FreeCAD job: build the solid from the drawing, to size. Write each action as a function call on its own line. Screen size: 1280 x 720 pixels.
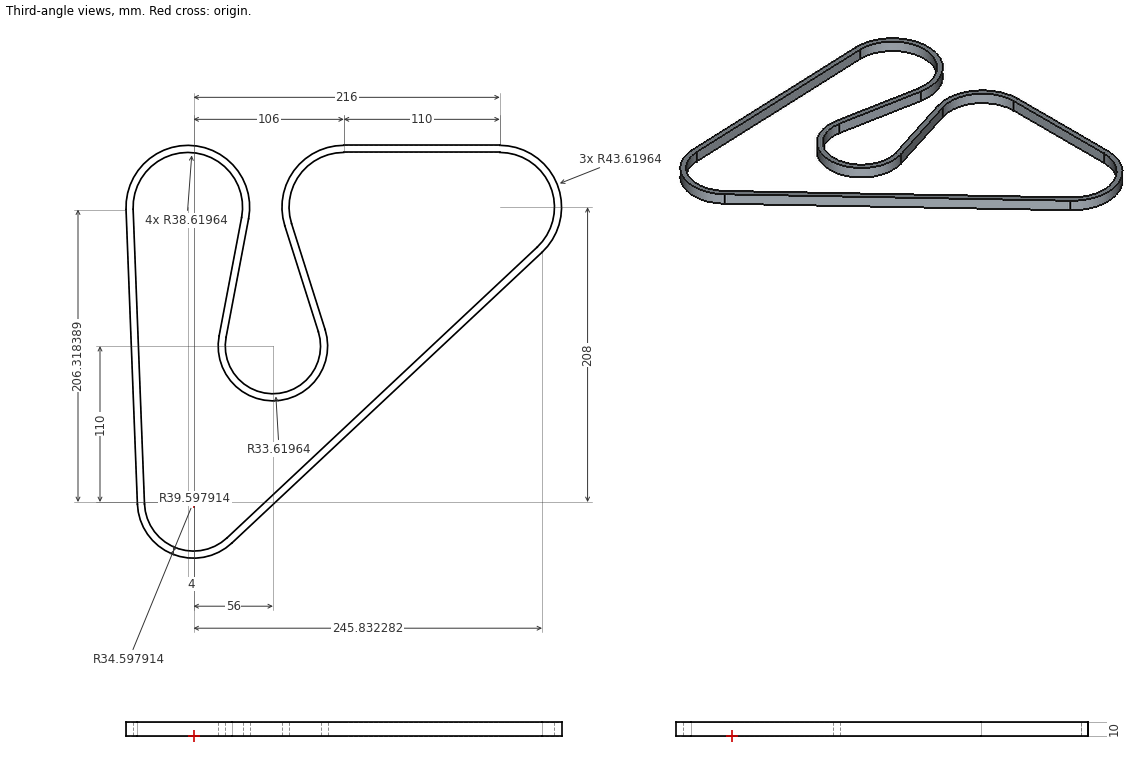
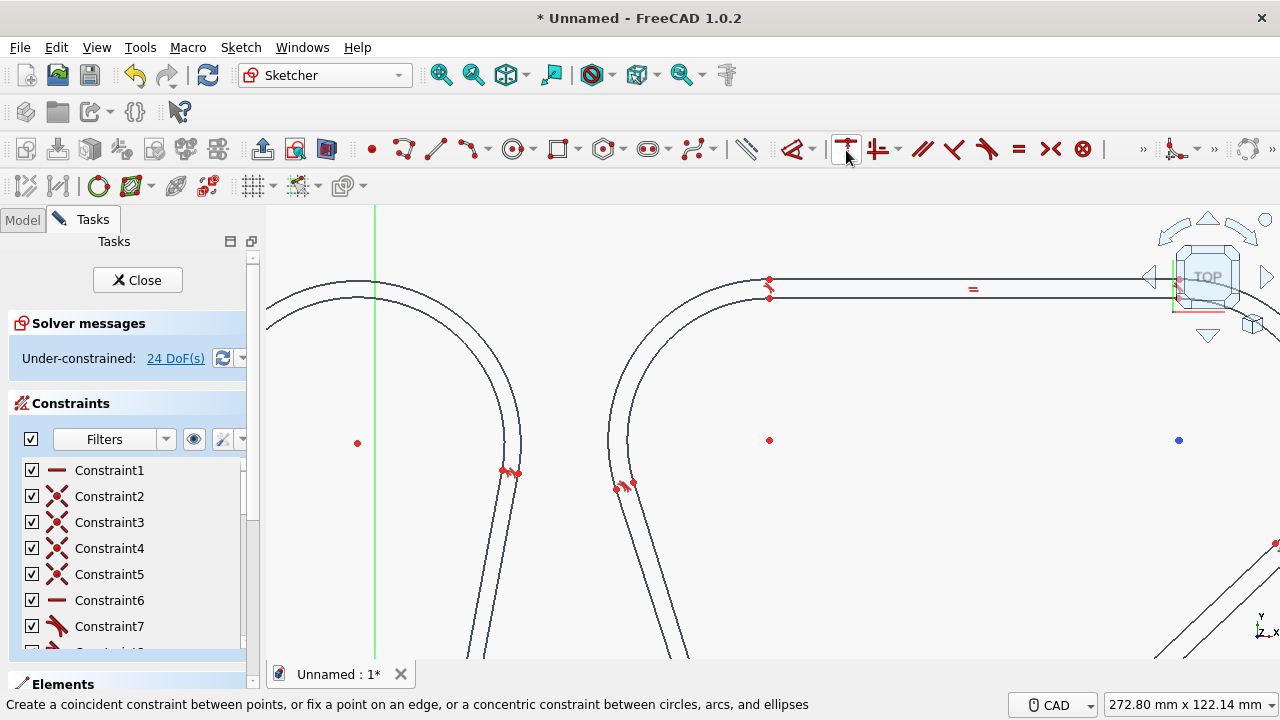
scroll(685, 308, down, 7)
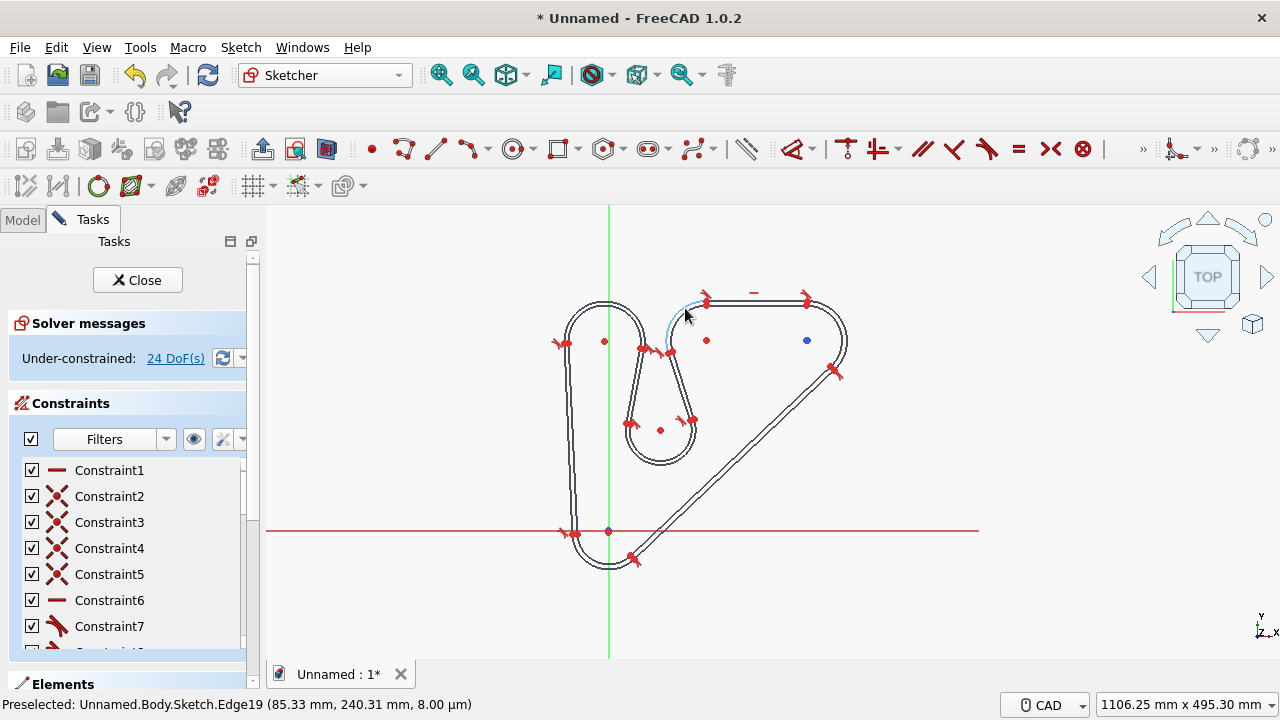
scroll(847, 345, up, 6)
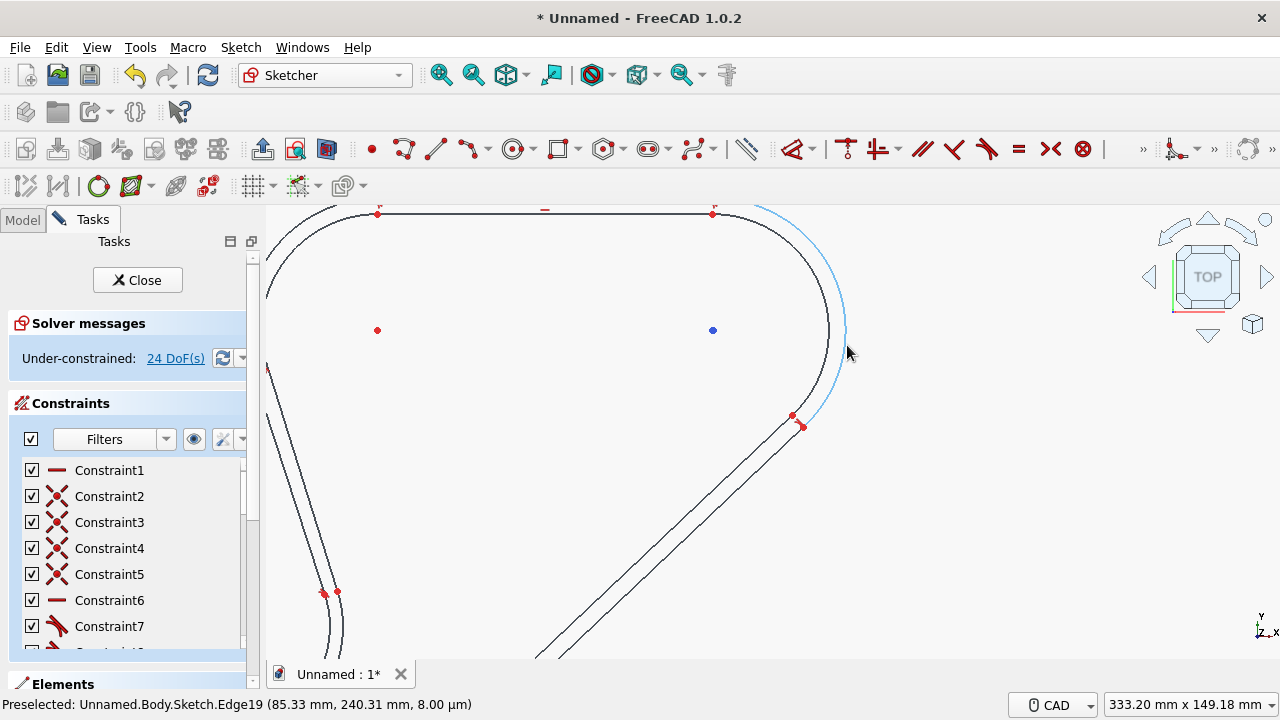
click(845, 344)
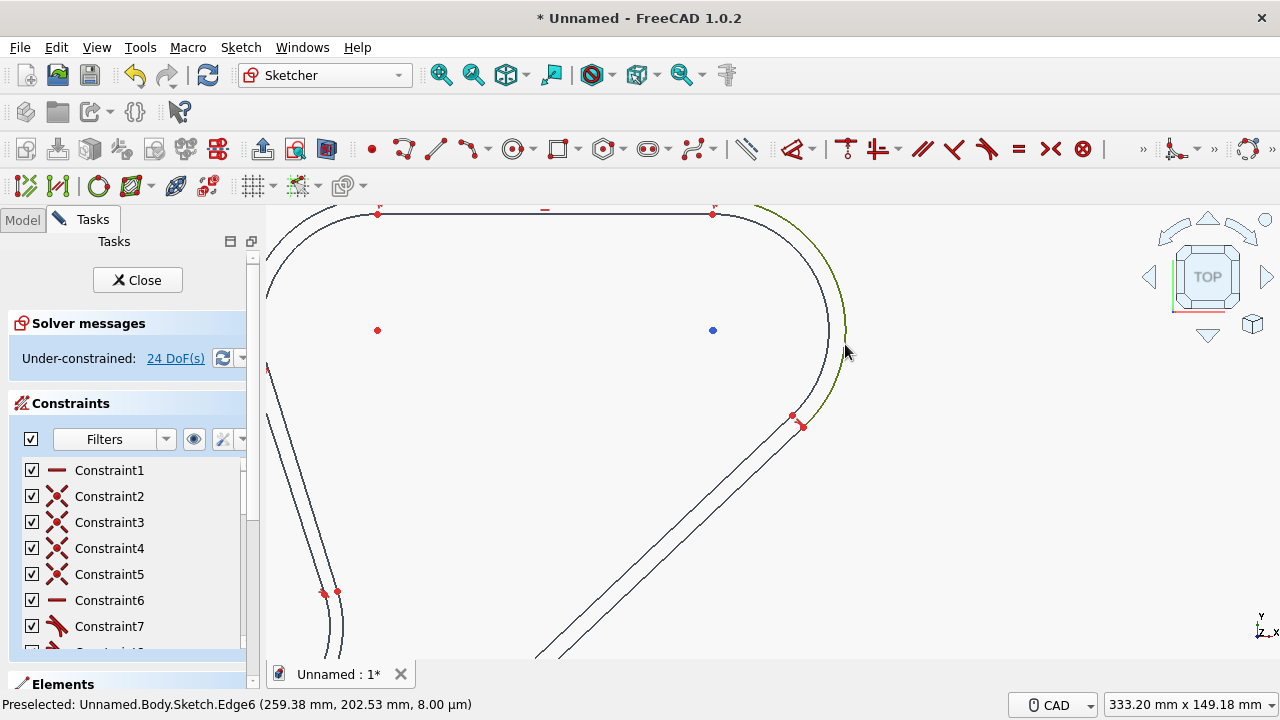
click(828, 342)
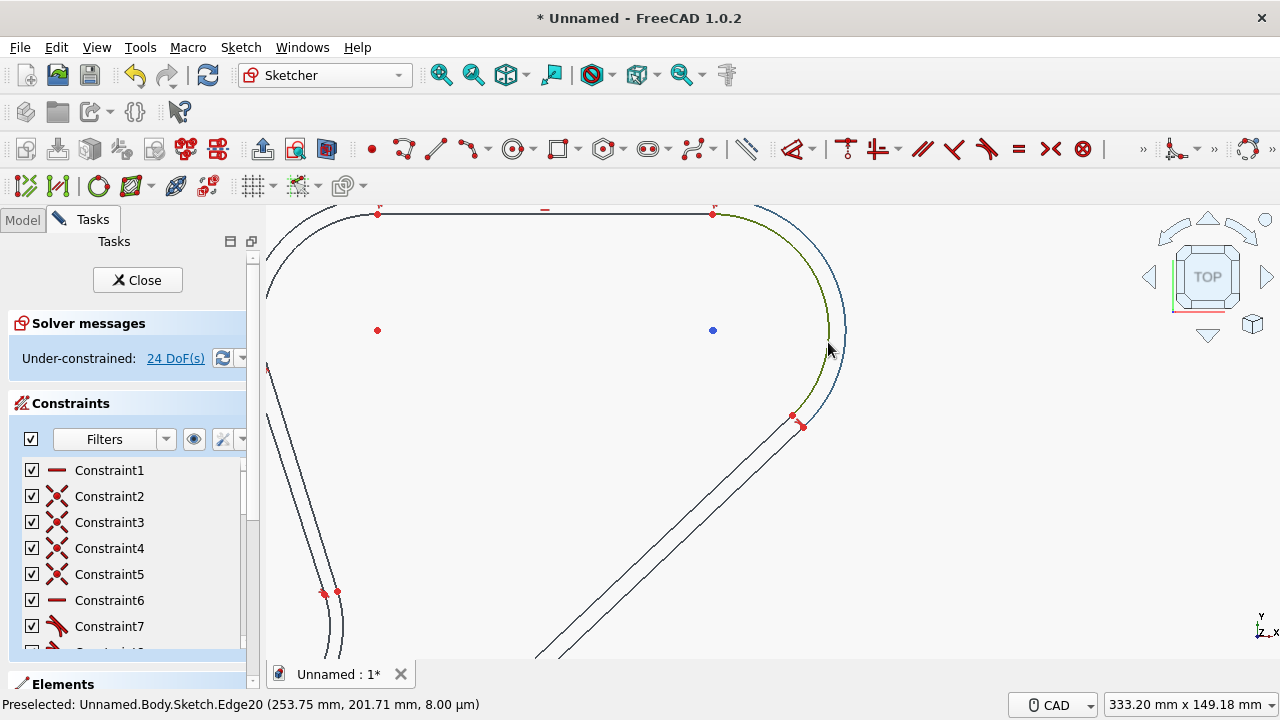
click(846, 150)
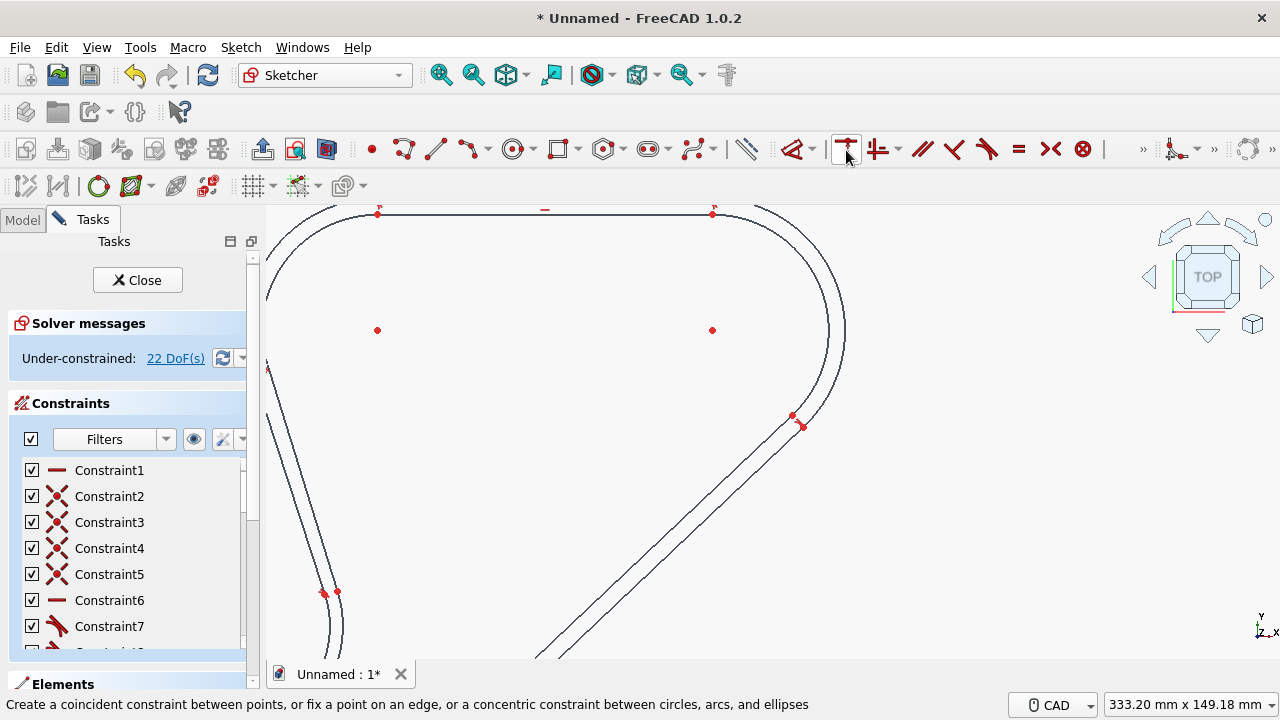
scroll(847, 345, down, 6)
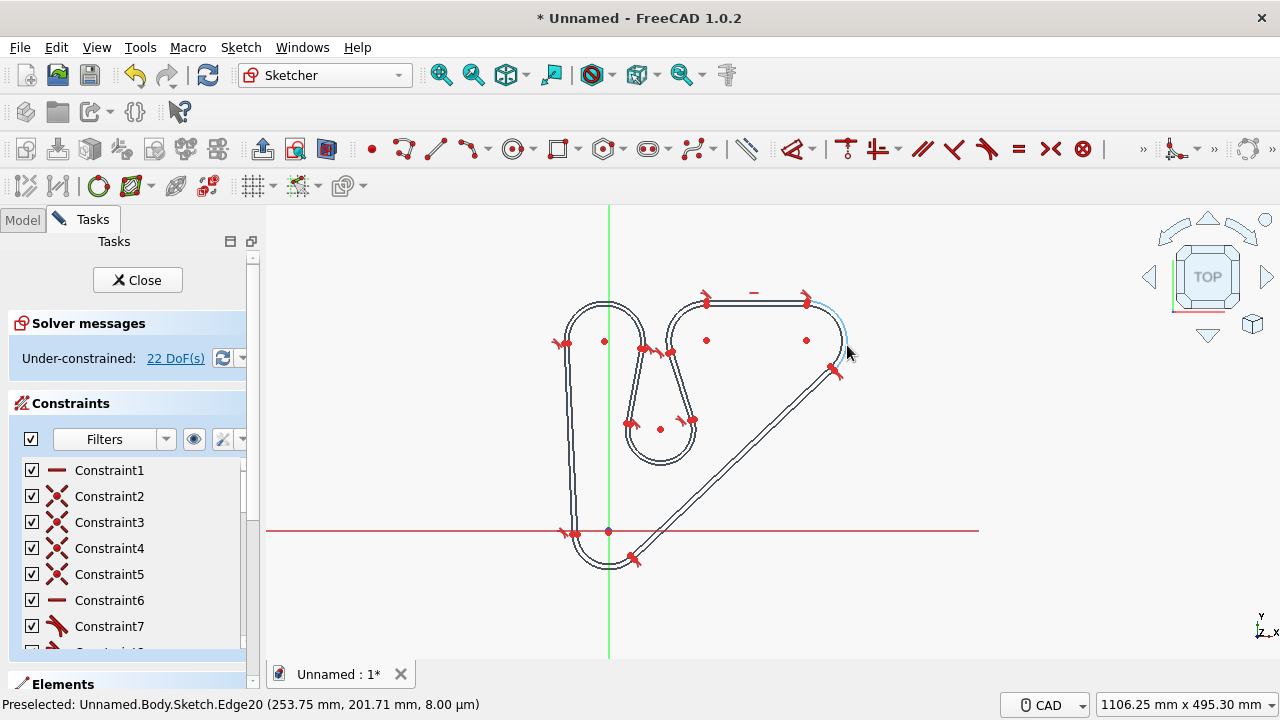
scroll(609, 532, up, 2)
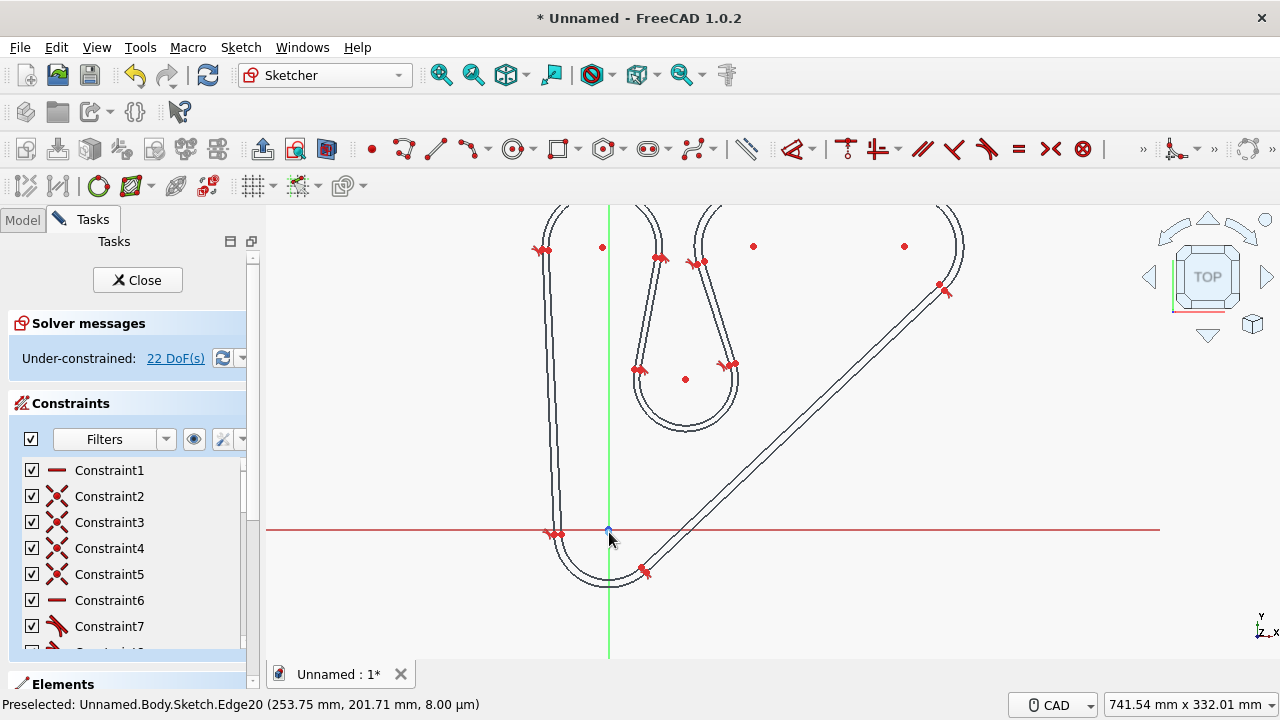
drag(599, 520, 619, 543)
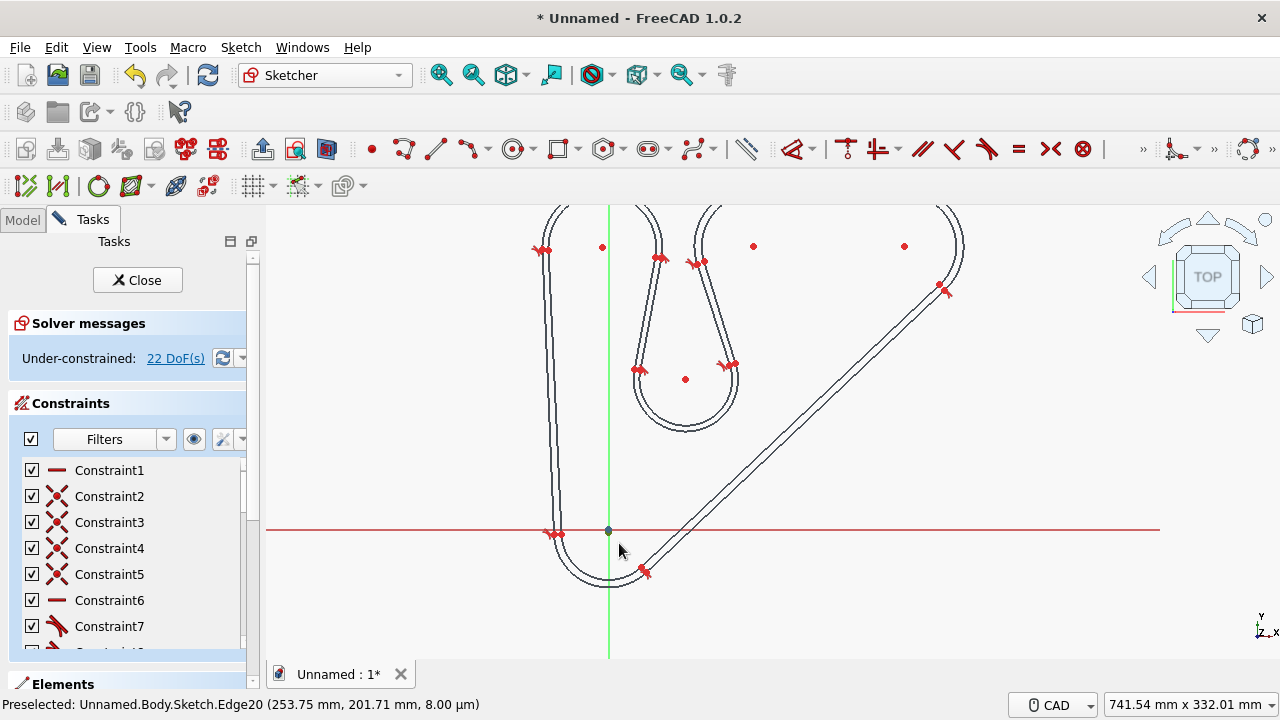
click(846, 150)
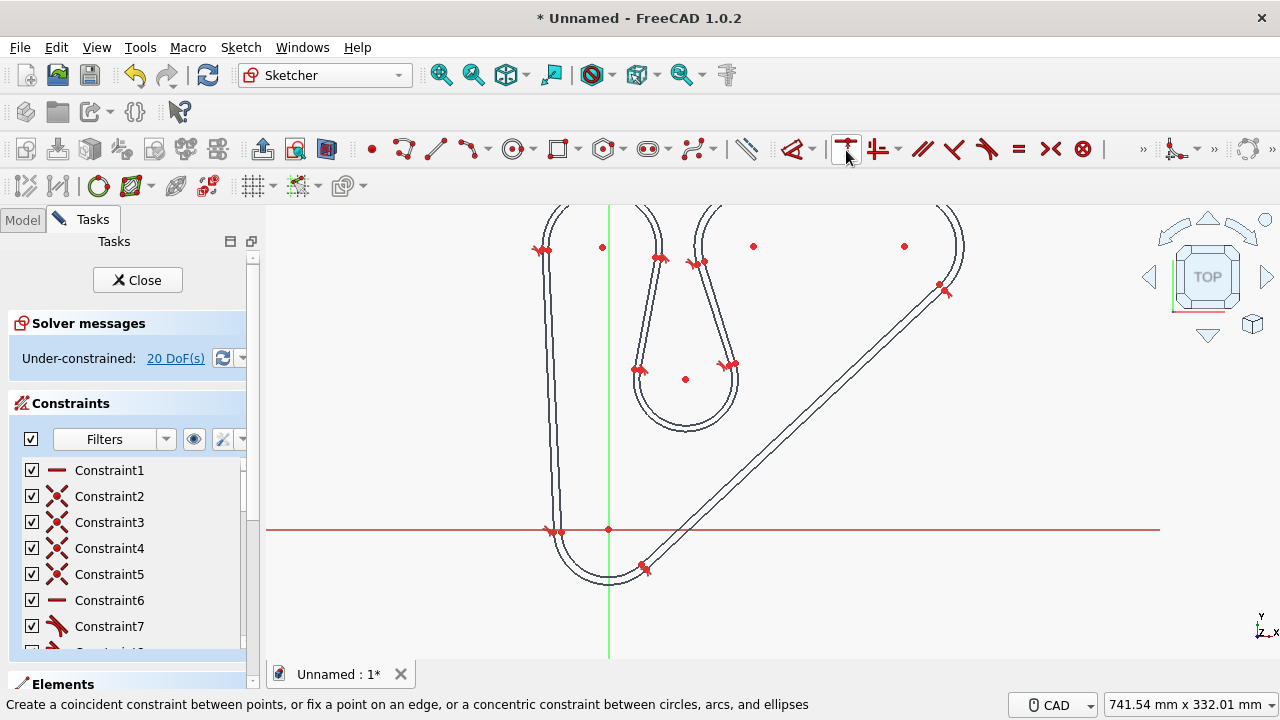
scroll(609, 532, down, 2)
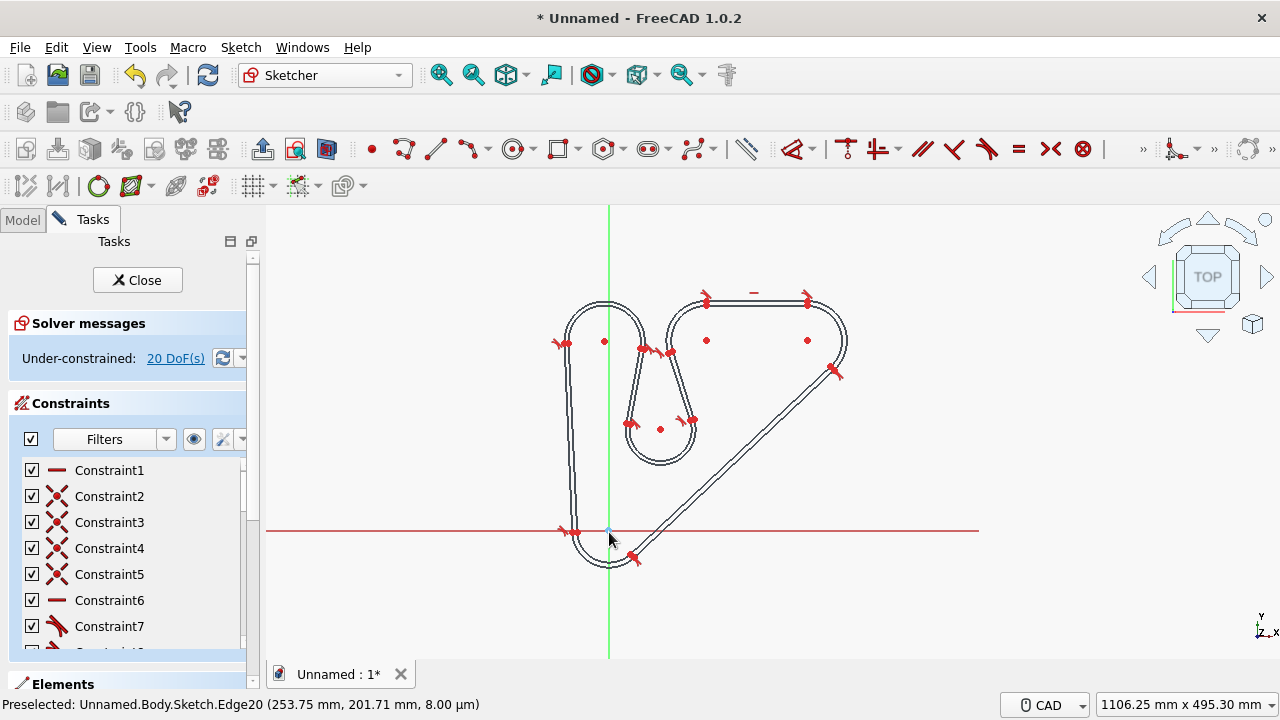
scroll(844, 326, up, 6)